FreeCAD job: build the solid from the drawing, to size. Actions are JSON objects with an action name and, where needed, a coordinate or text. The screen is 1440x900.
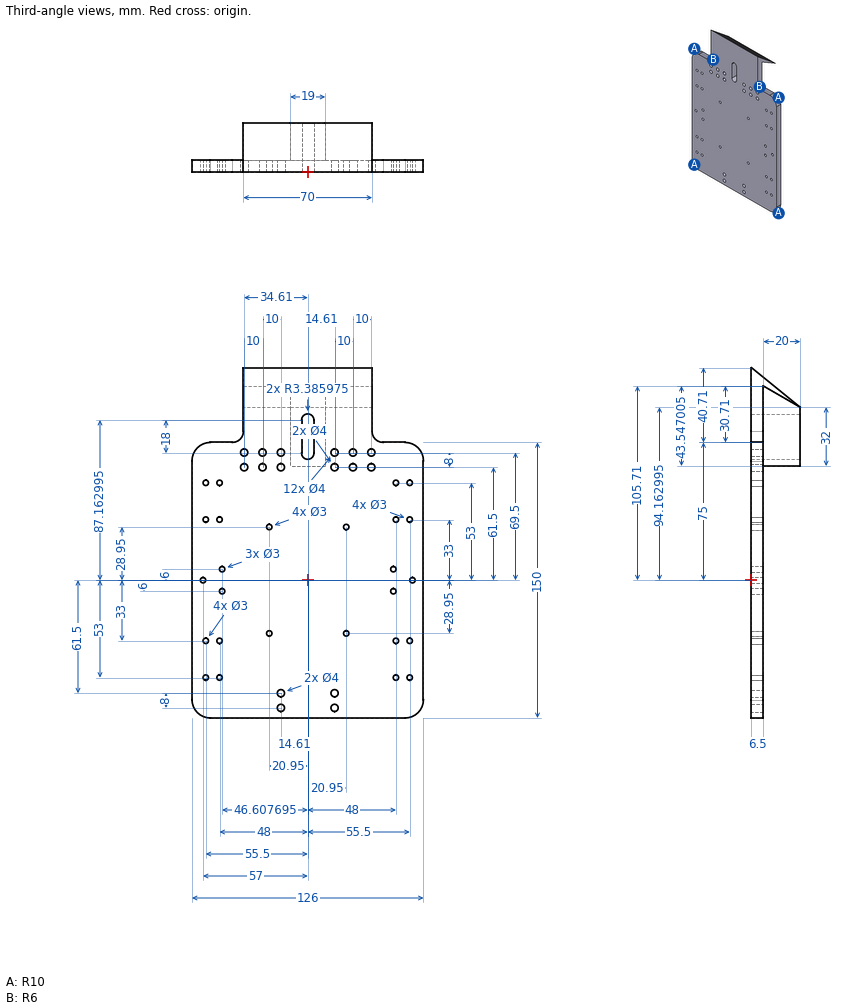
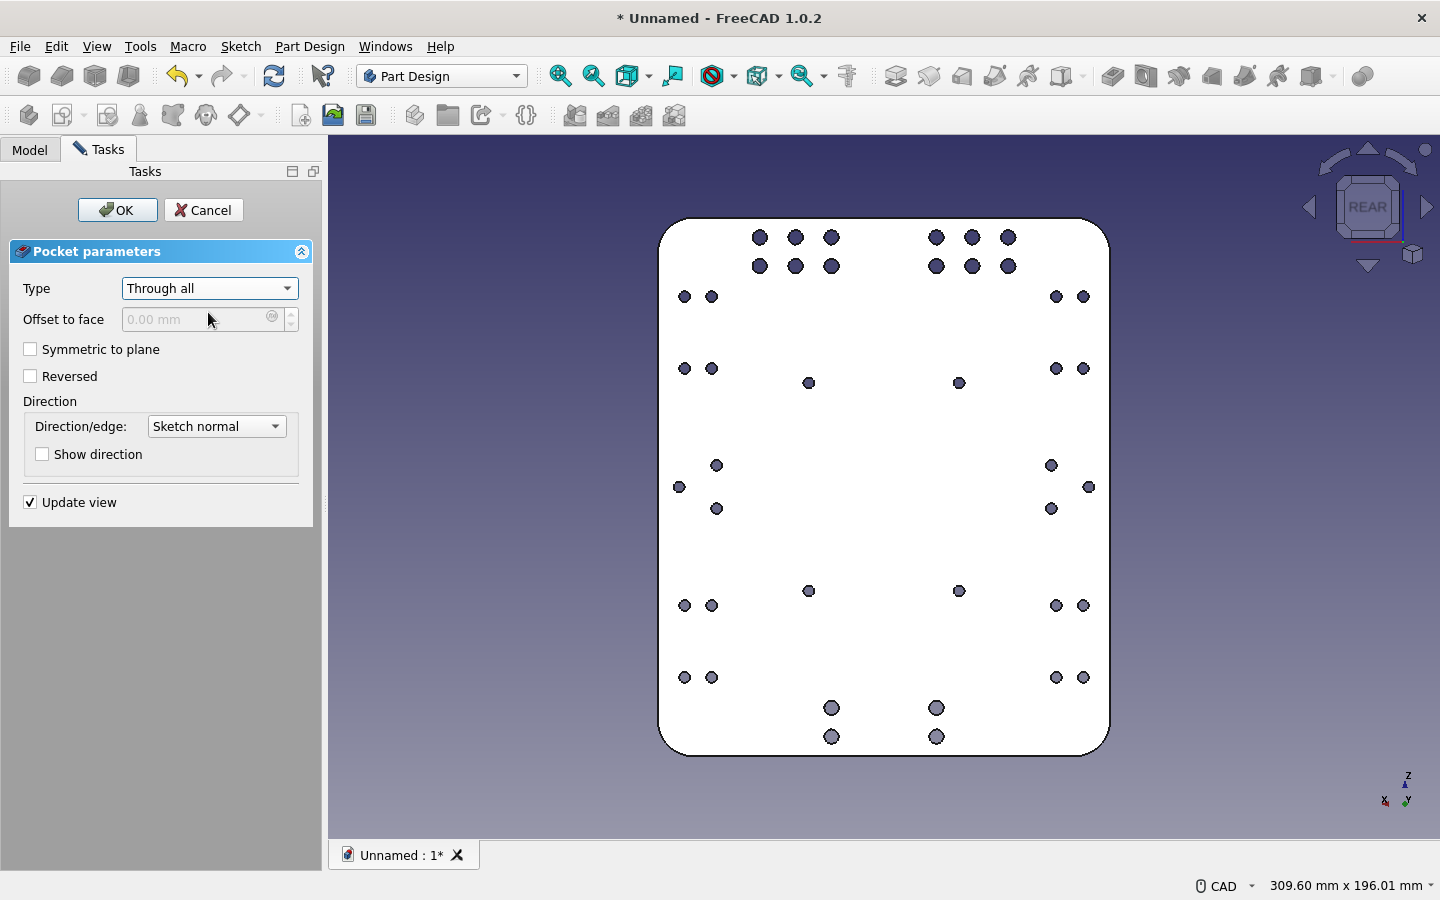
{"action": "left_click", "coordinate": [118, 210]}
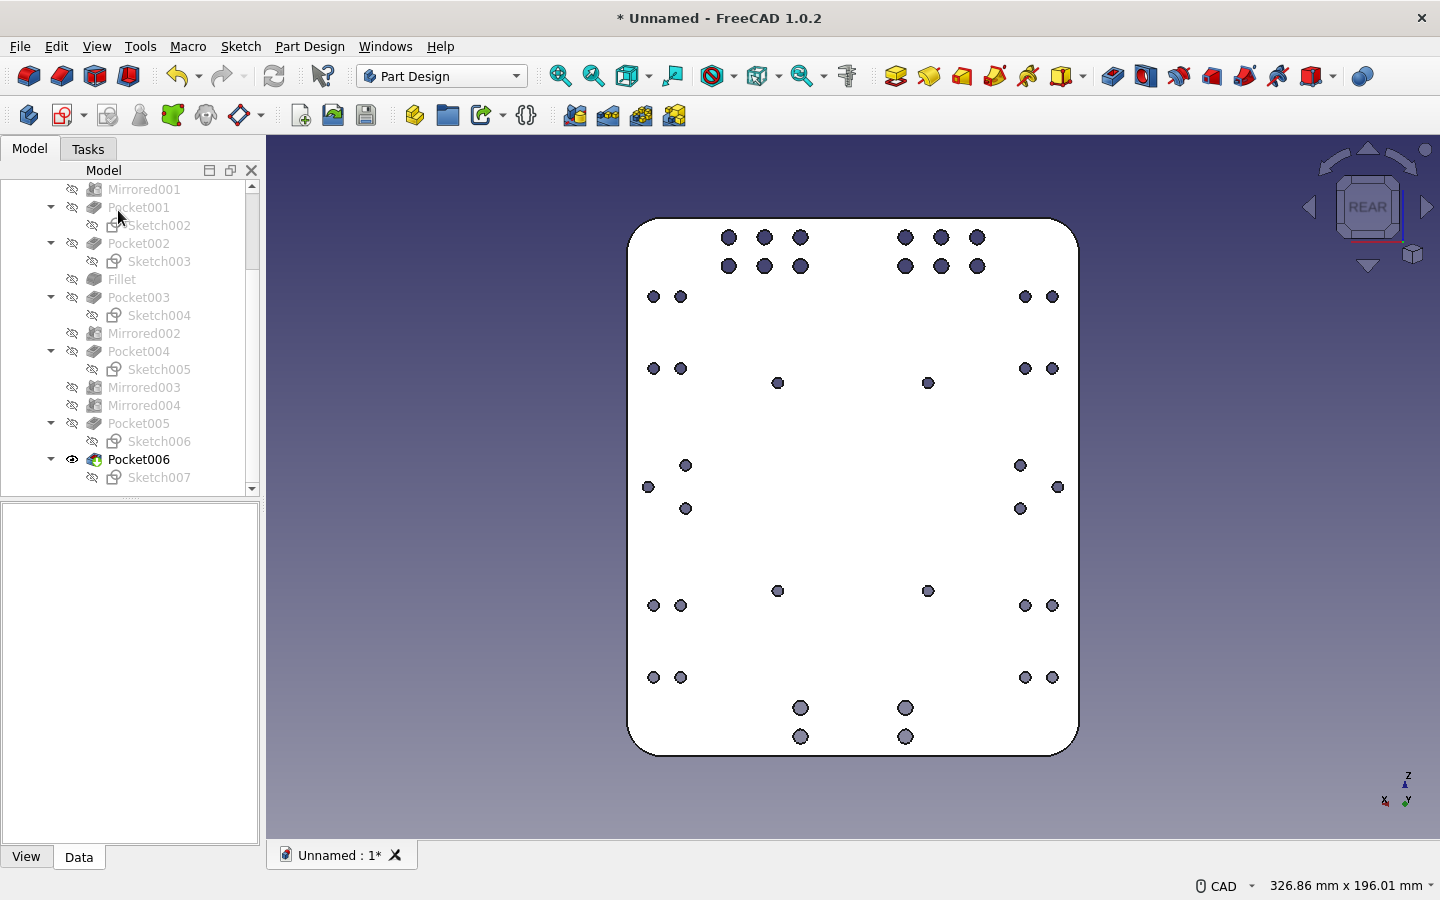
{"action": "left_click", "coordinate": [62, 116]}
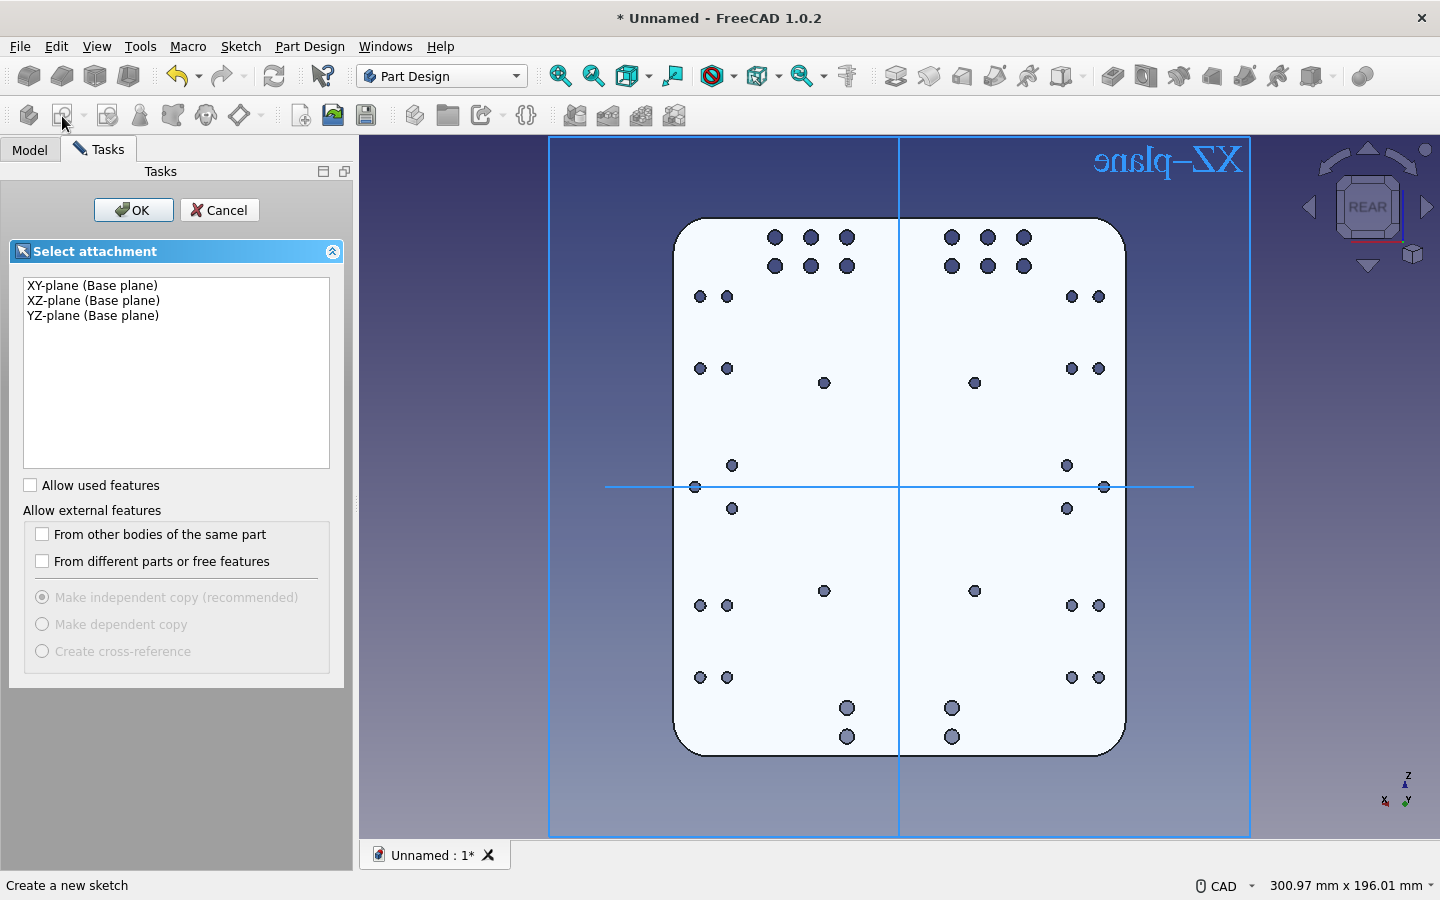
{"action": "left_click", "coordinate": [84, 316]}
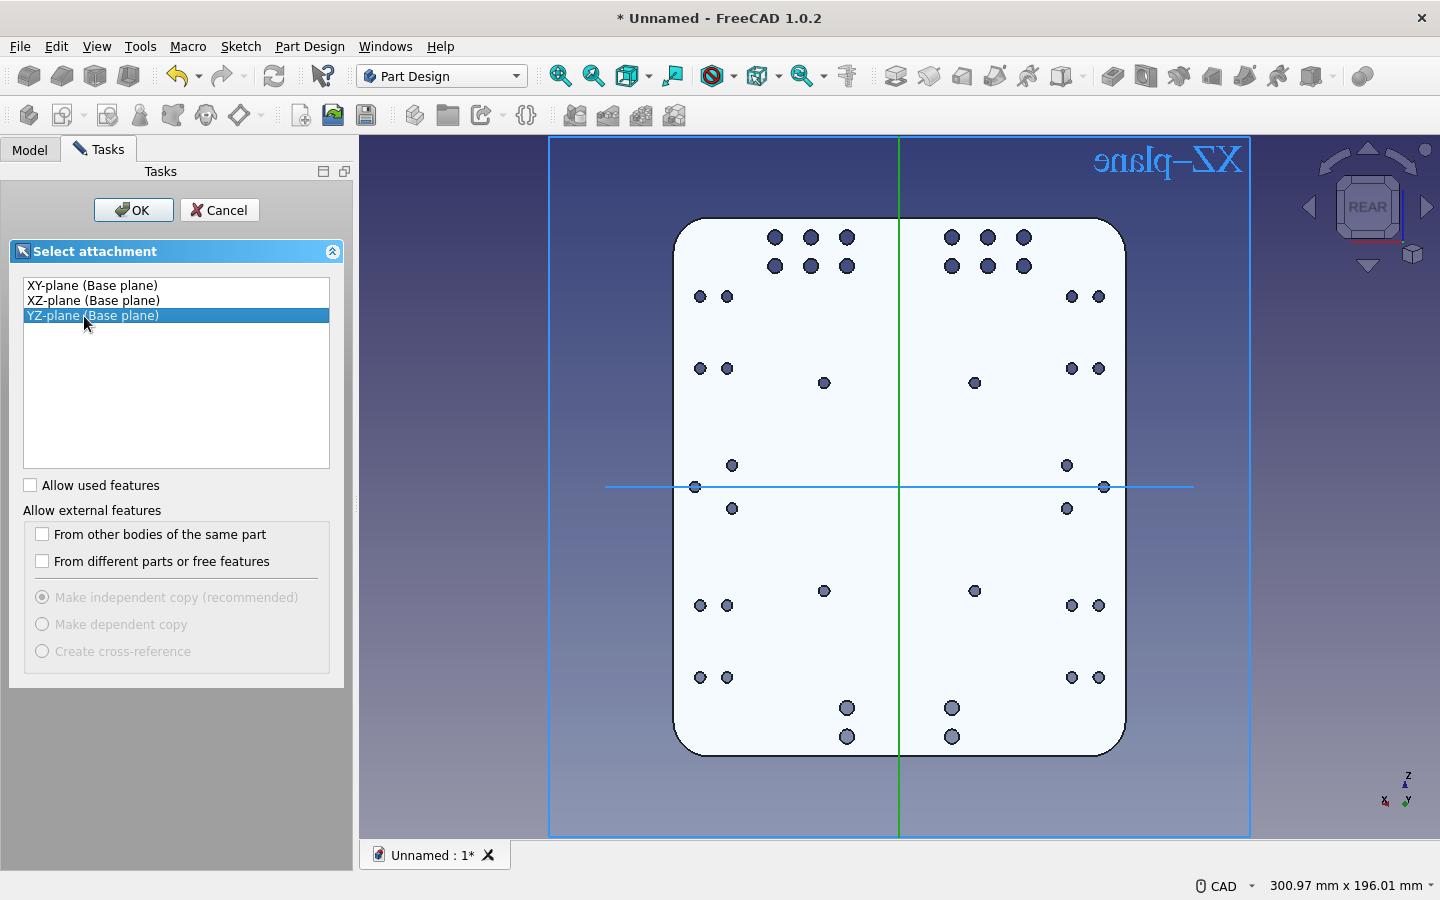
{"action": "left_click", "coordinate": [134, 210]}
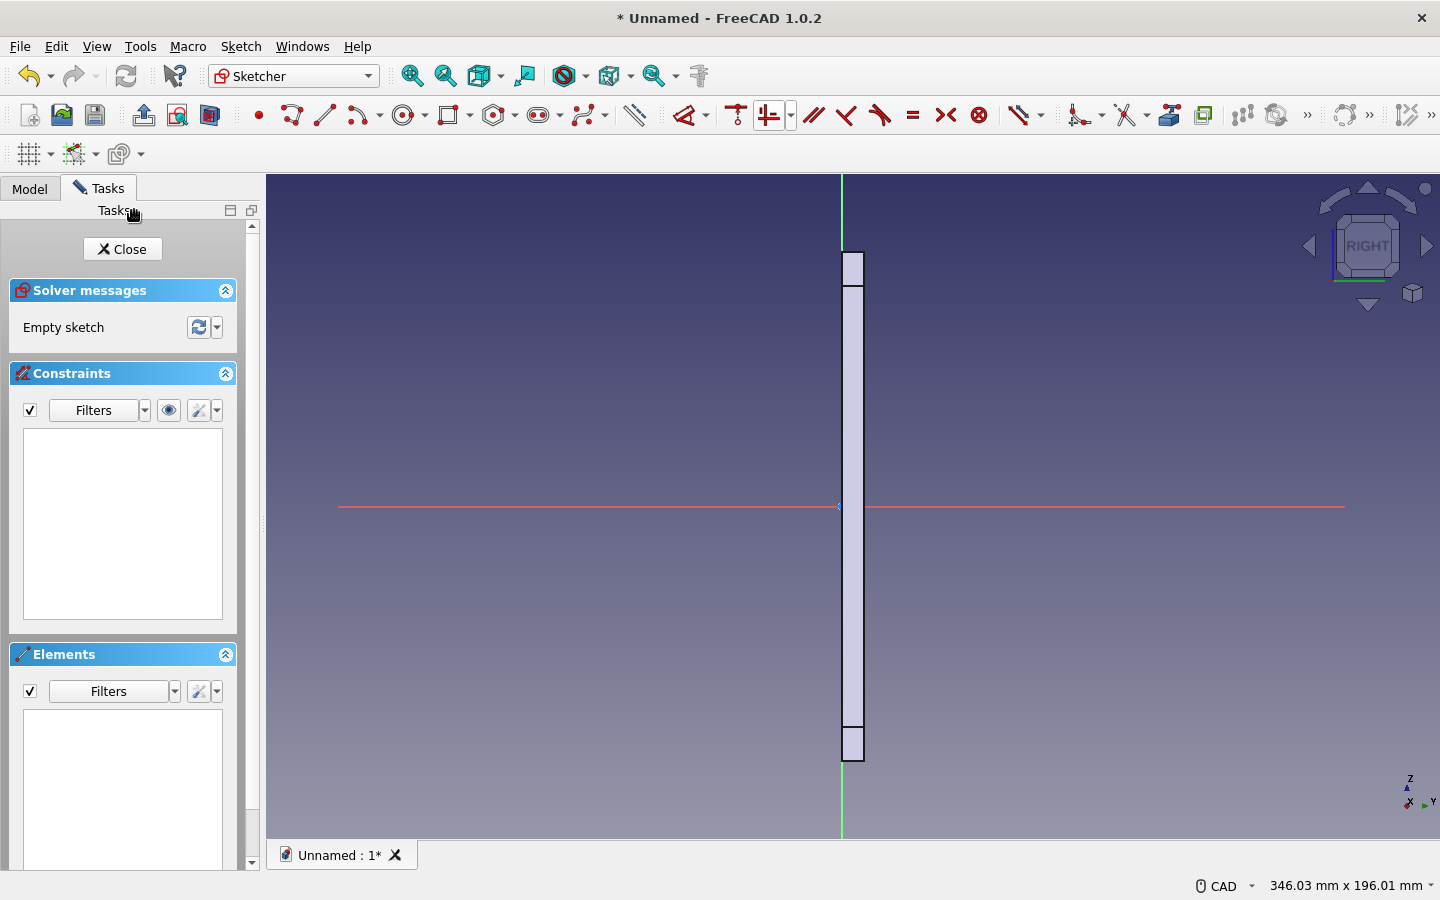
{"action": "key", "text": "q s"}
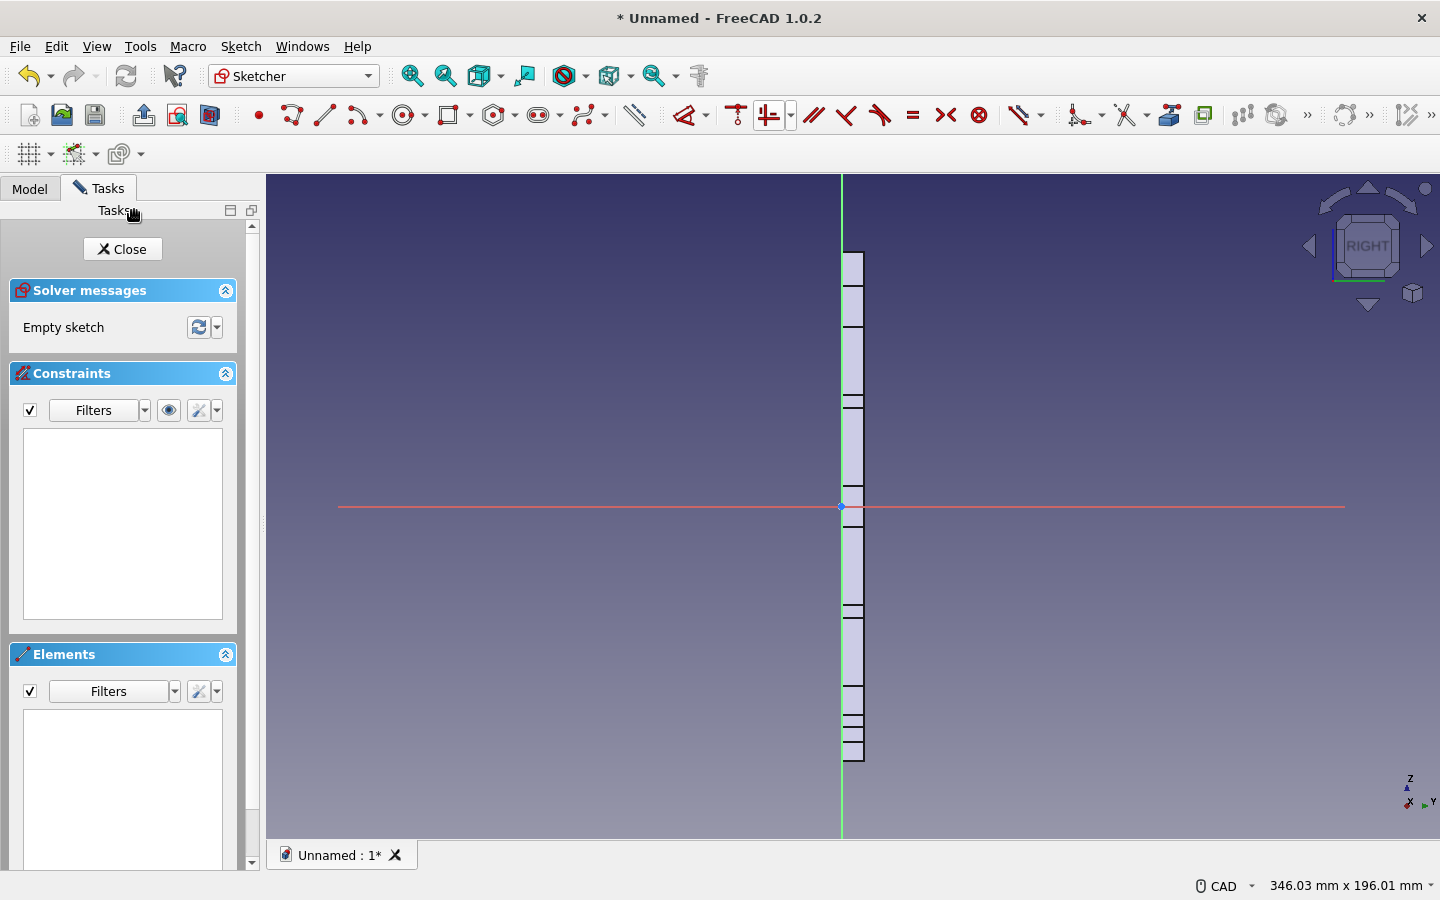
{"action": "scroll", "coordinate": [784, 506], "scroll_direction": "down", "scroll_amount": 5}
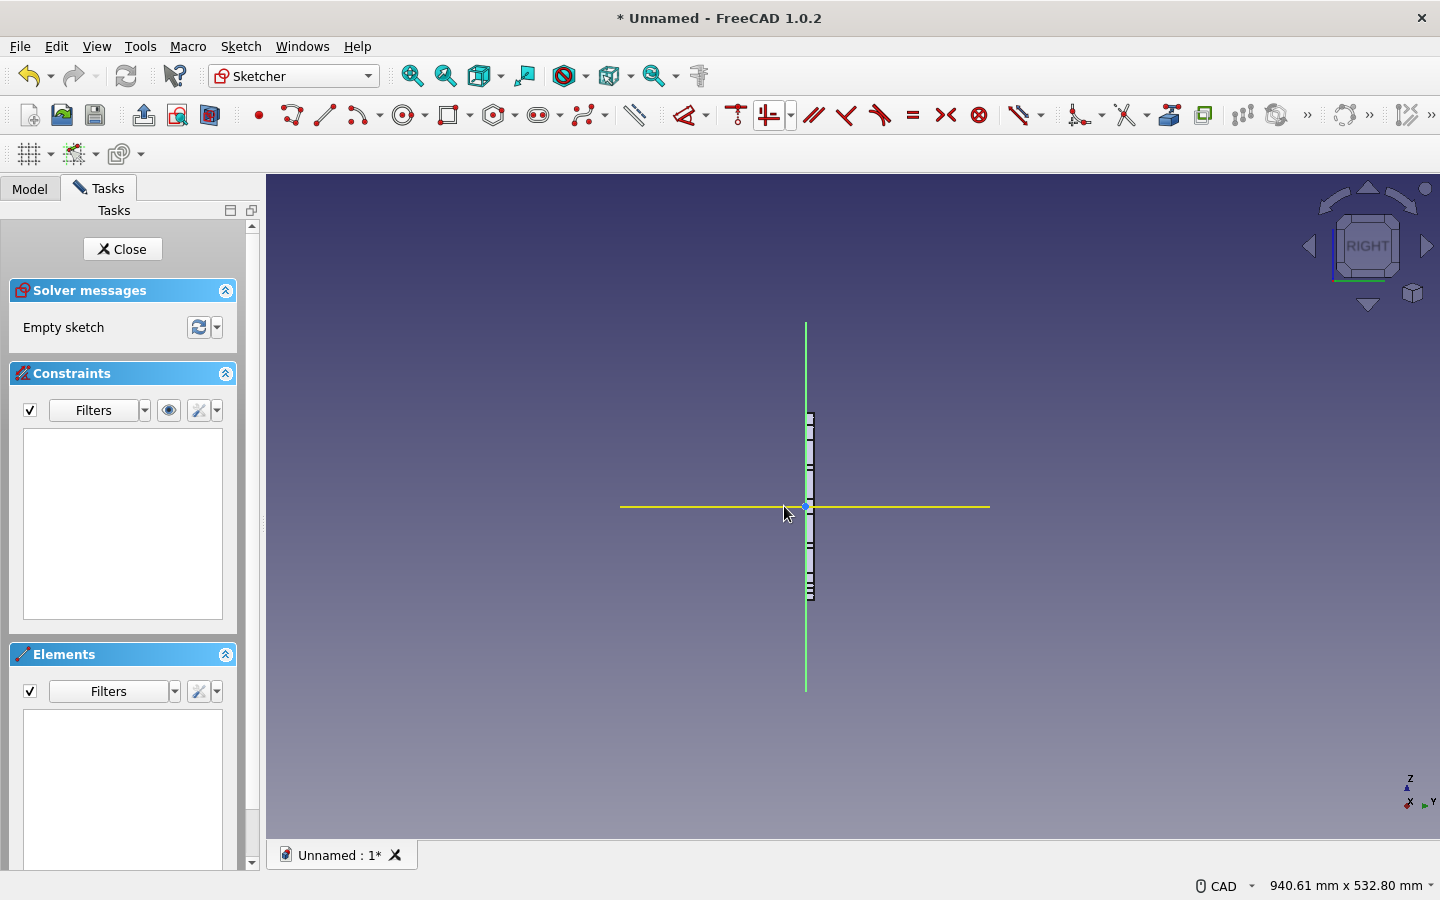
{"action": "scroll", "coordinate": [827, 373], "scroll_direction": "up", "scroll_amount": 11}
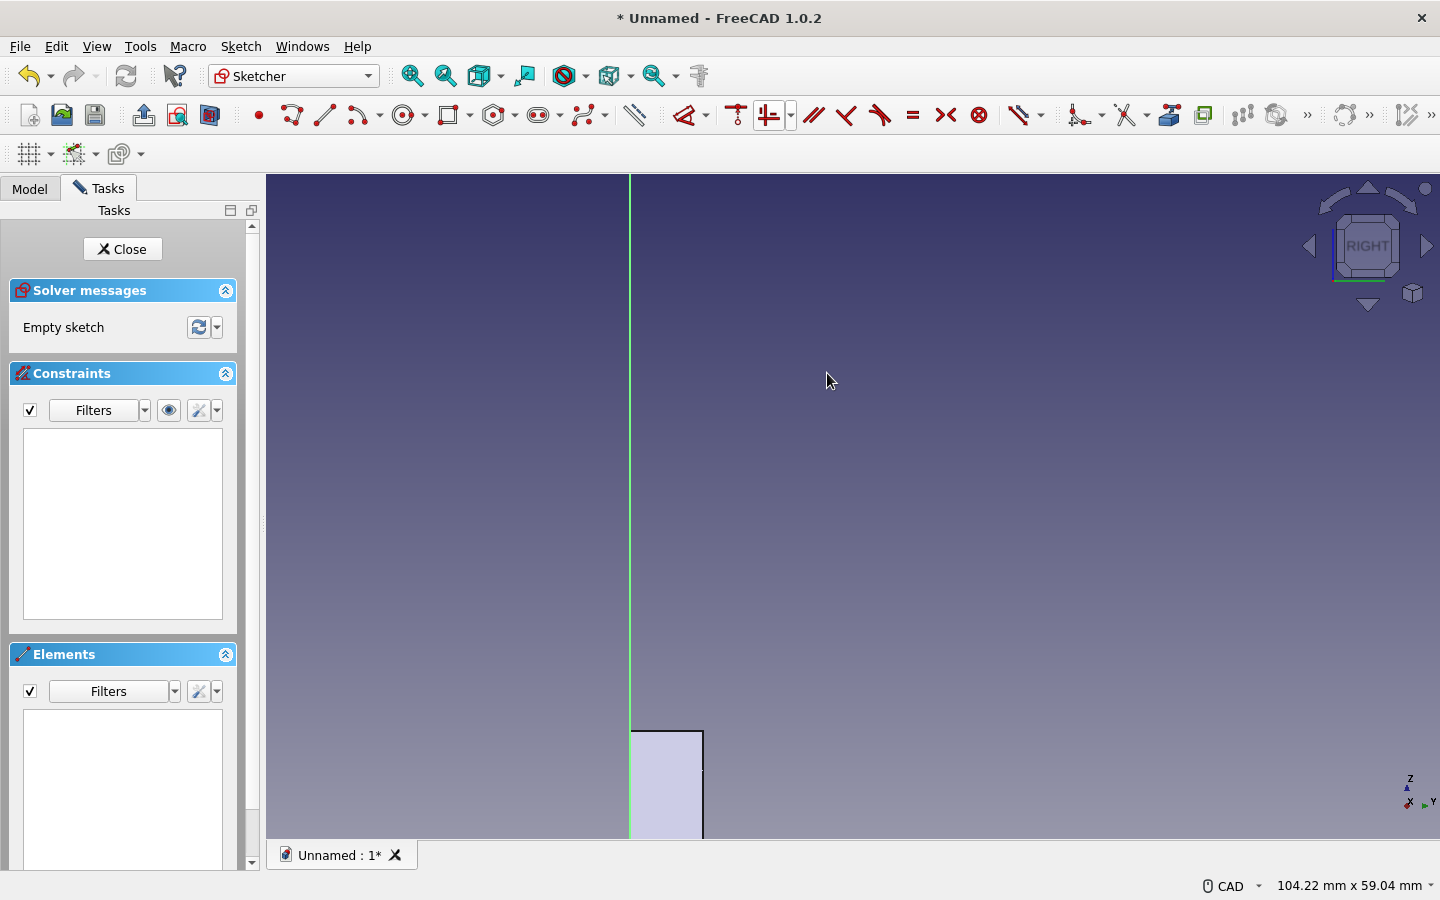
{"action": "left_click", "coordinate": [292, 116]}